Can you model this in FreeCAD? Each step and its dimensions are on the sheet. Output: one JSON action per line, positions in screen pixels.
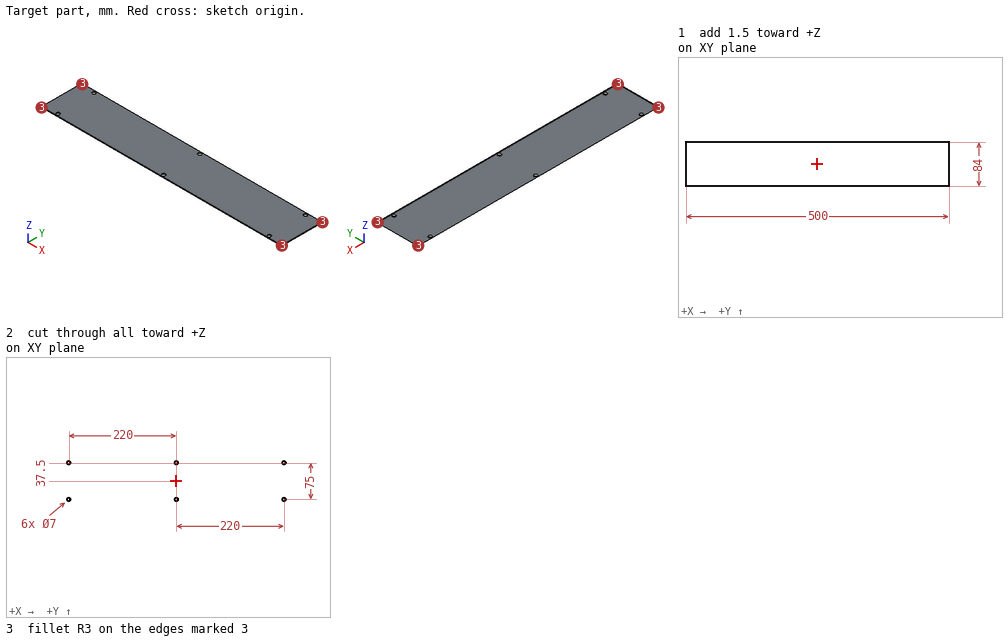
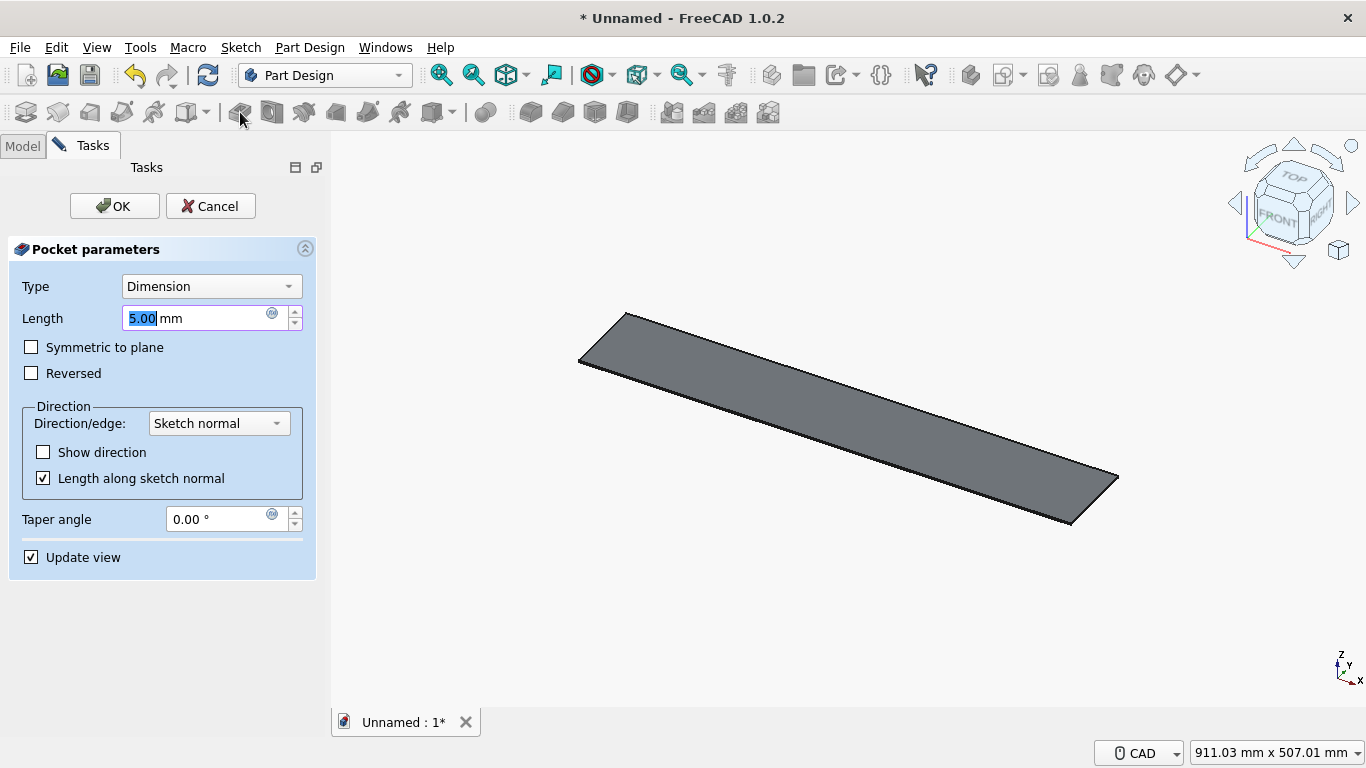
{"action": "left_click", "coordinate": [212, 286]}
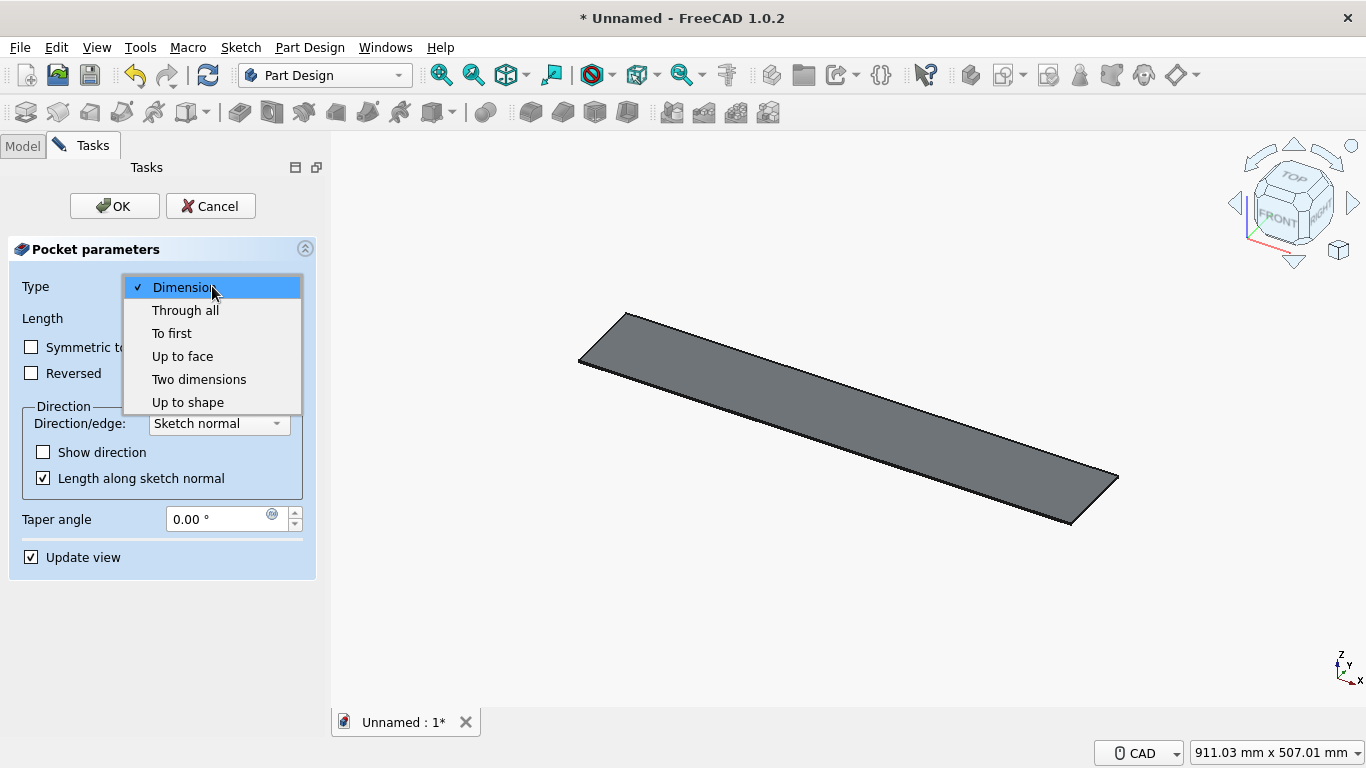
{"action": "left_click", "coordinate": [212, 310]}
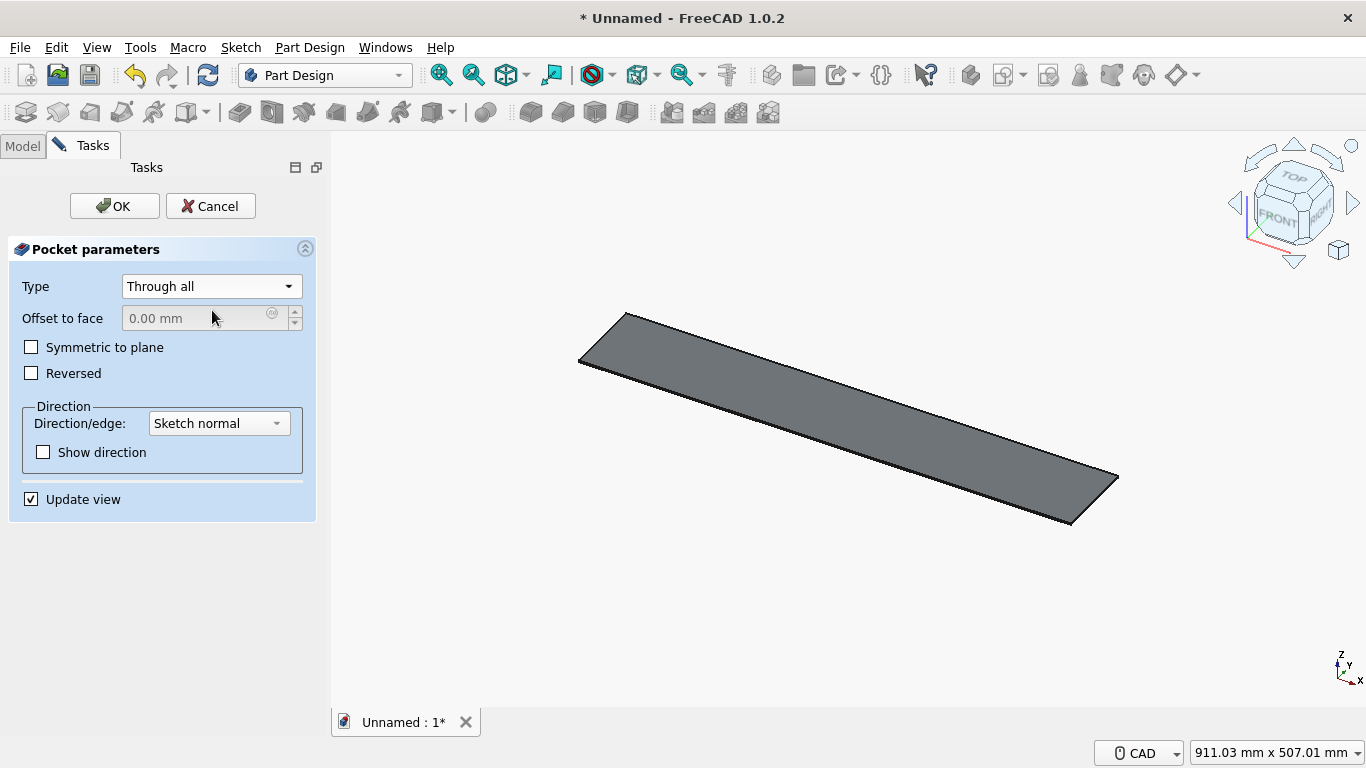
{"action": "left_click", "coordinate": [30, 373]}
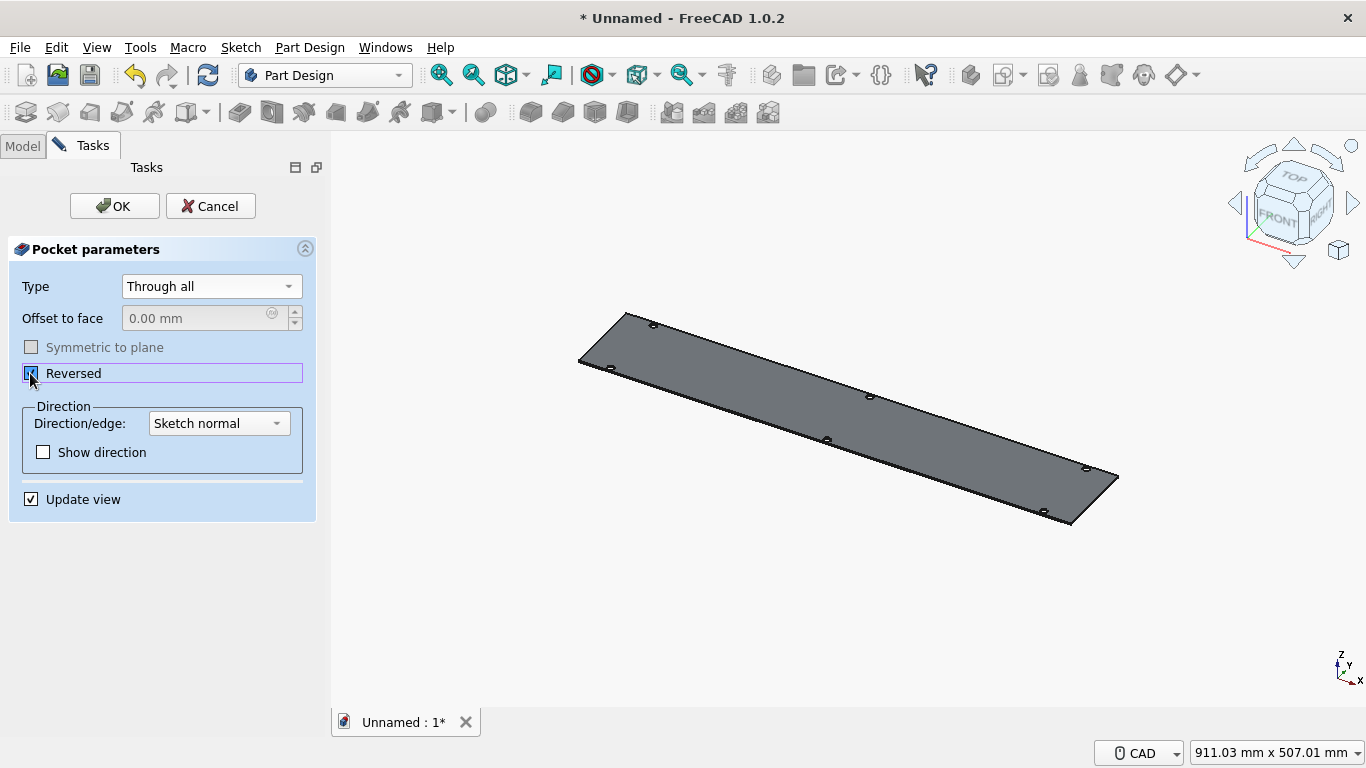
{"action": "left_click", "coordinate": [115, 206]}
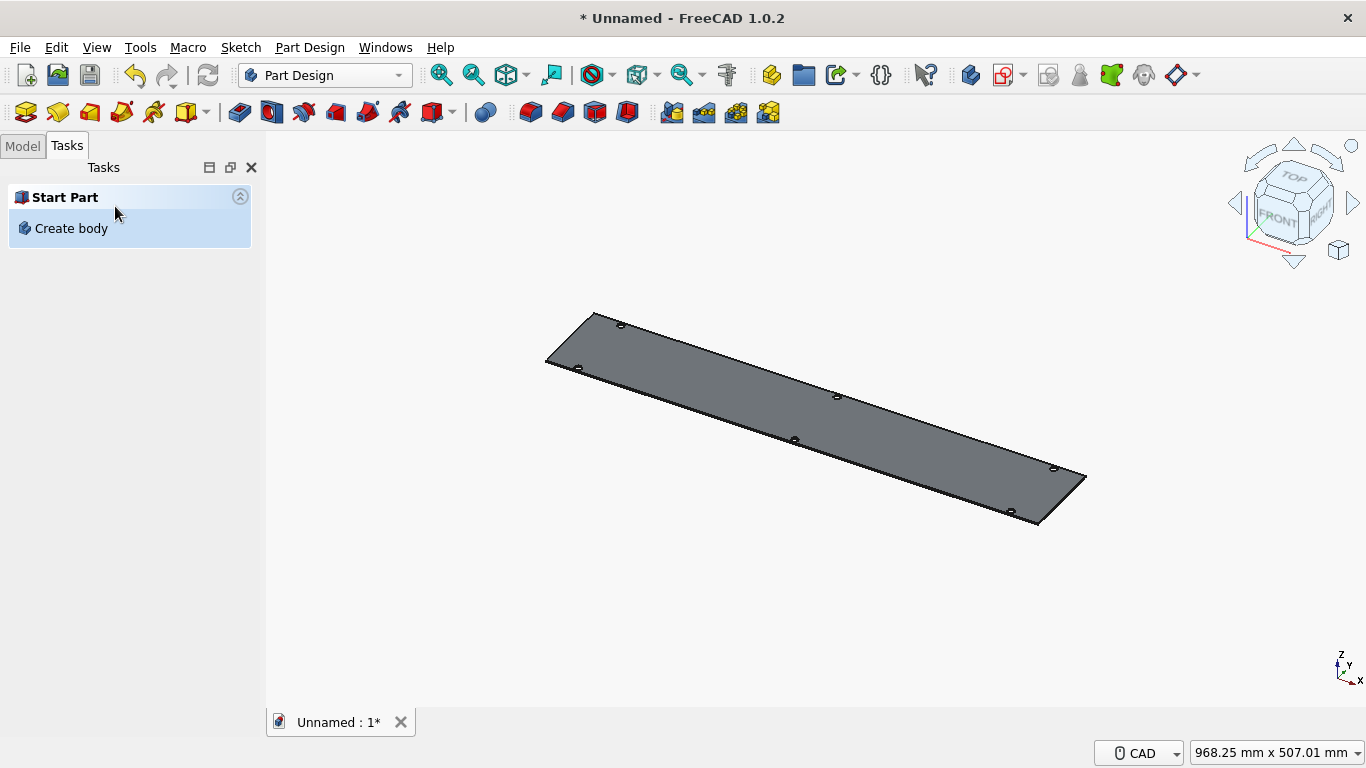
{"action": "scroll", "coordinate": [1038, 523], "scroll_direction": "up", "scroll_amount": 15}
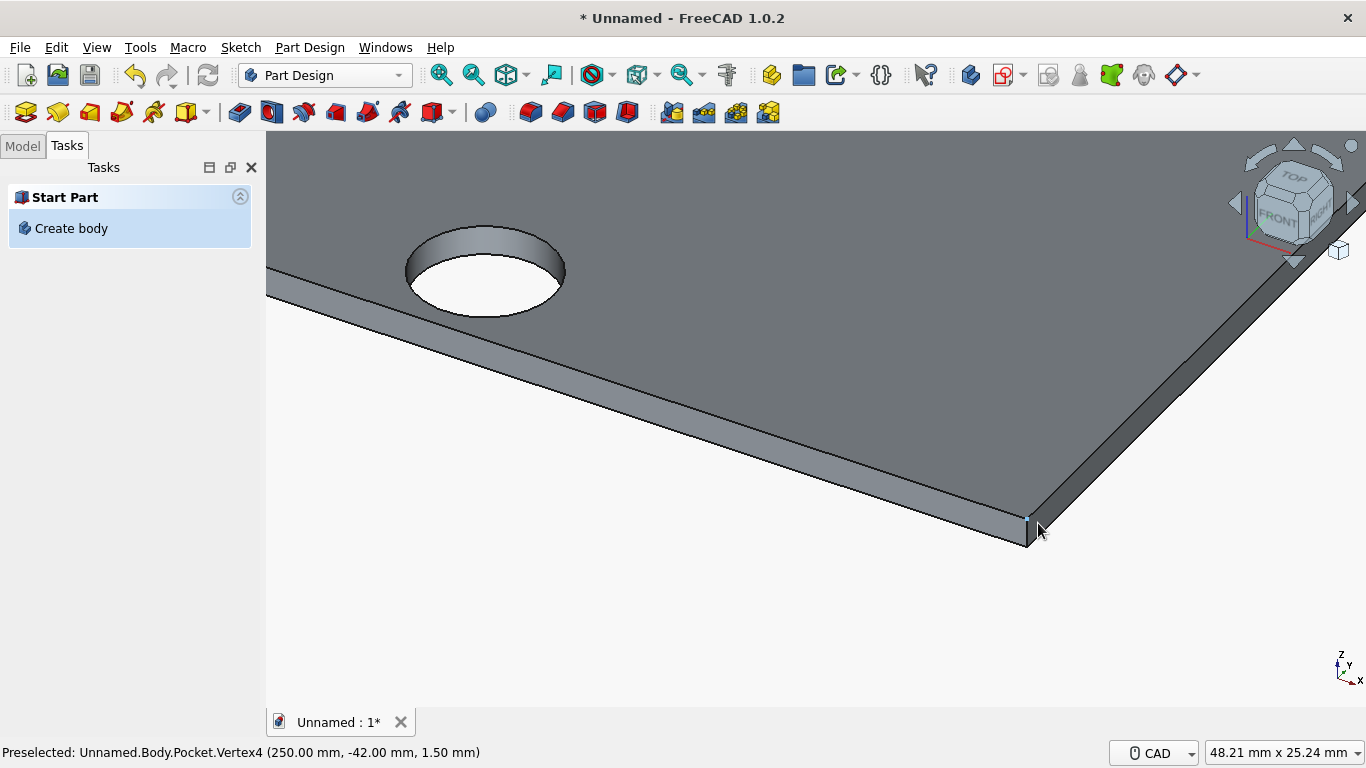
{"action": "left_click", "coordinate": [1027, 532]}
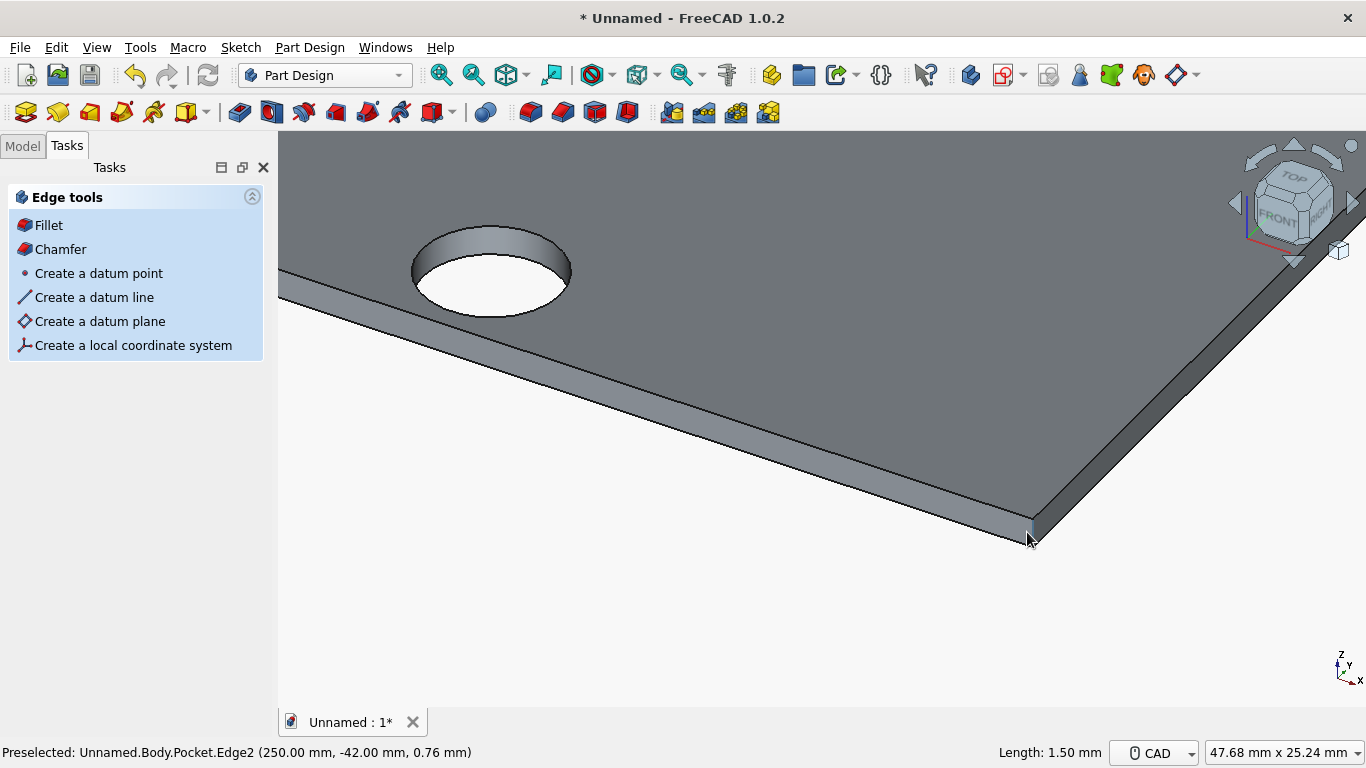
{"action": "left_click", "coordinate": [442, 76]}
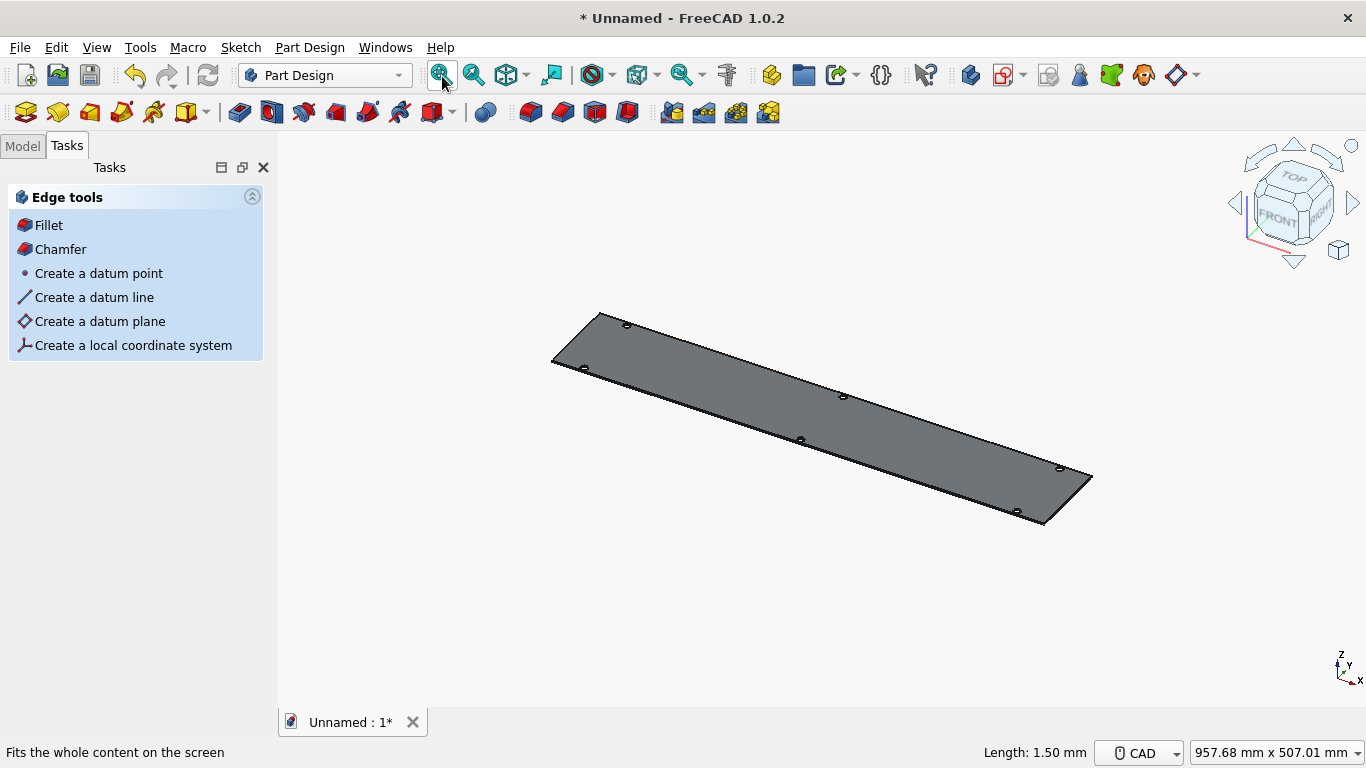
{"action": "key", "text": "0"}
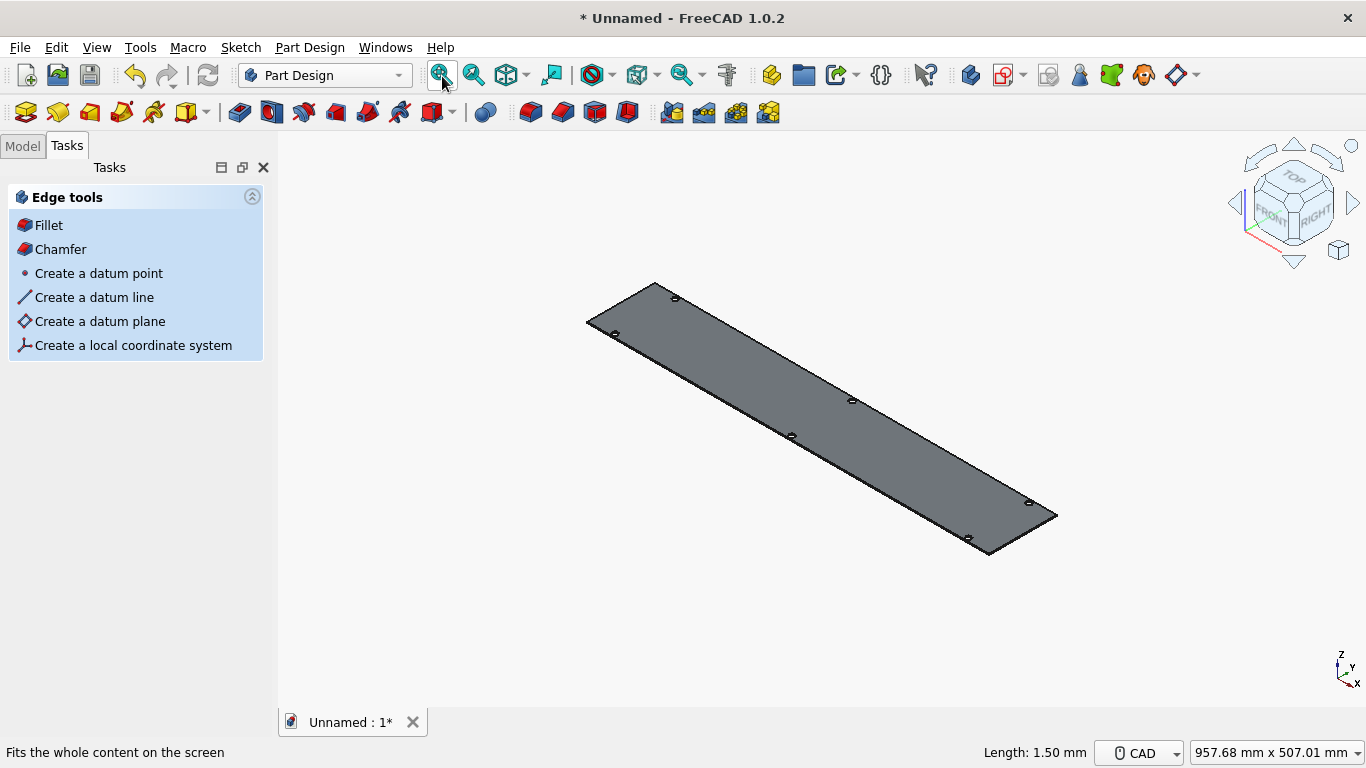
{"action": "scroll", "coordinate": [587, 322], "scroll_direction": "up", "scroll_amount": 15}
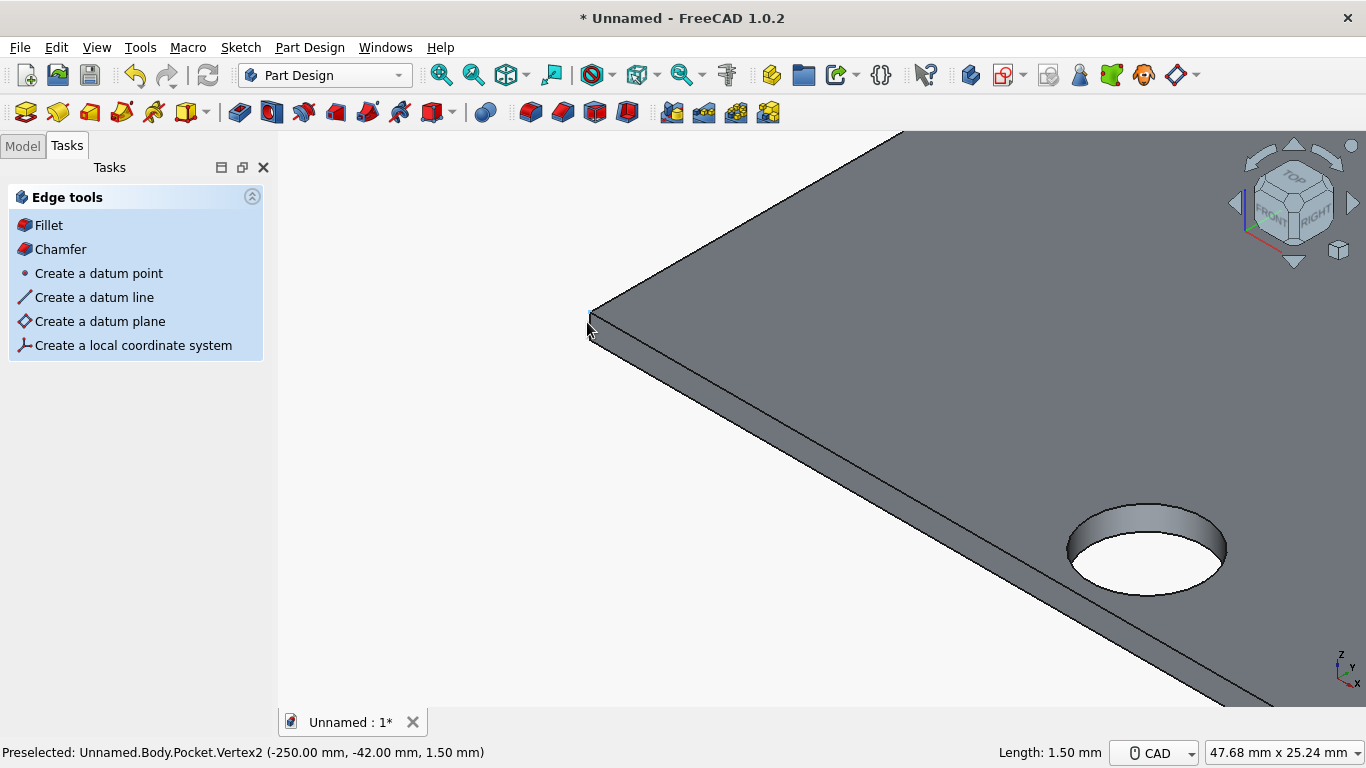
{"action": "left_click", "coordinate": [442, 76]}